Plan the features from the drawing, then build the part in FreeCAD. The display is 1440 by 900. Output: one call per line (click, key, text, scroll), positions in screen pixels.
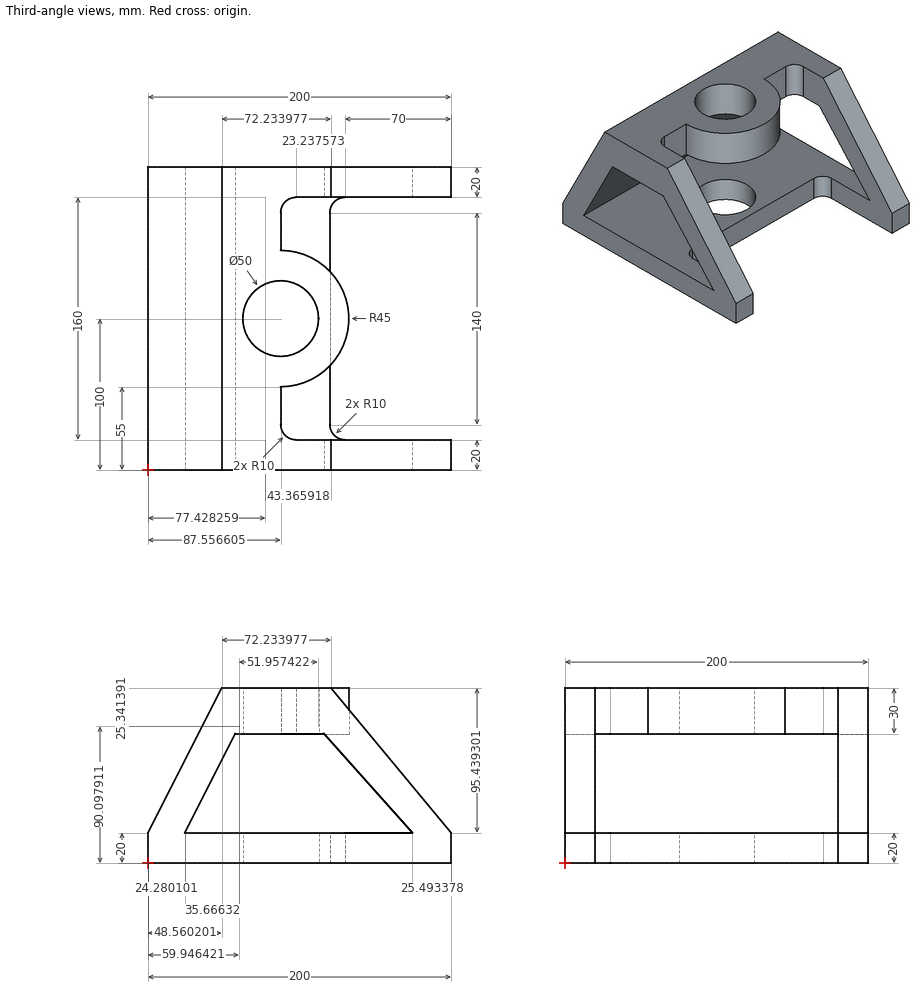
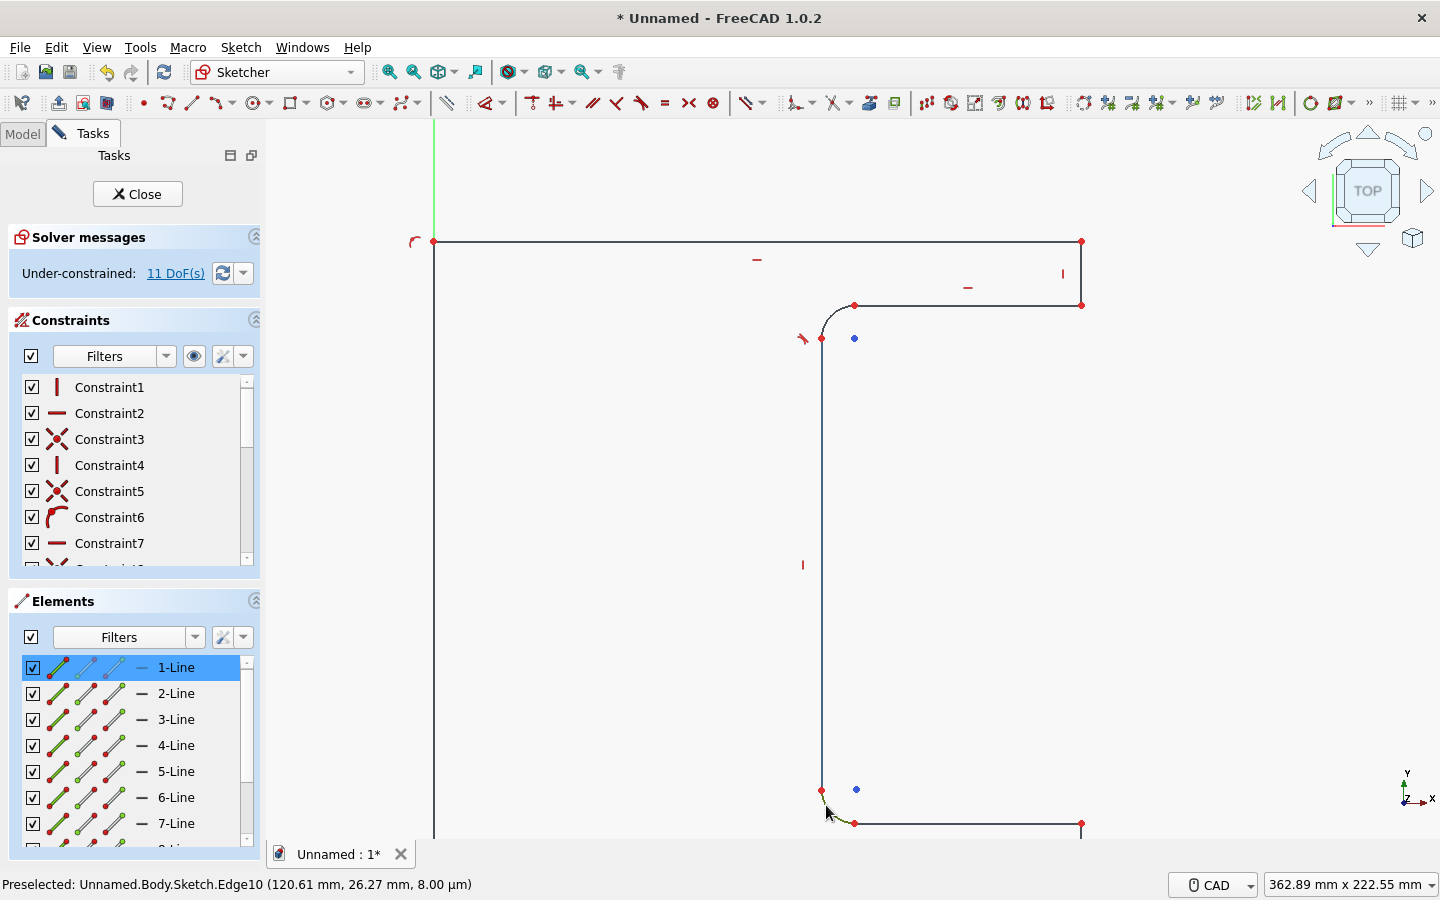
click(642, 104)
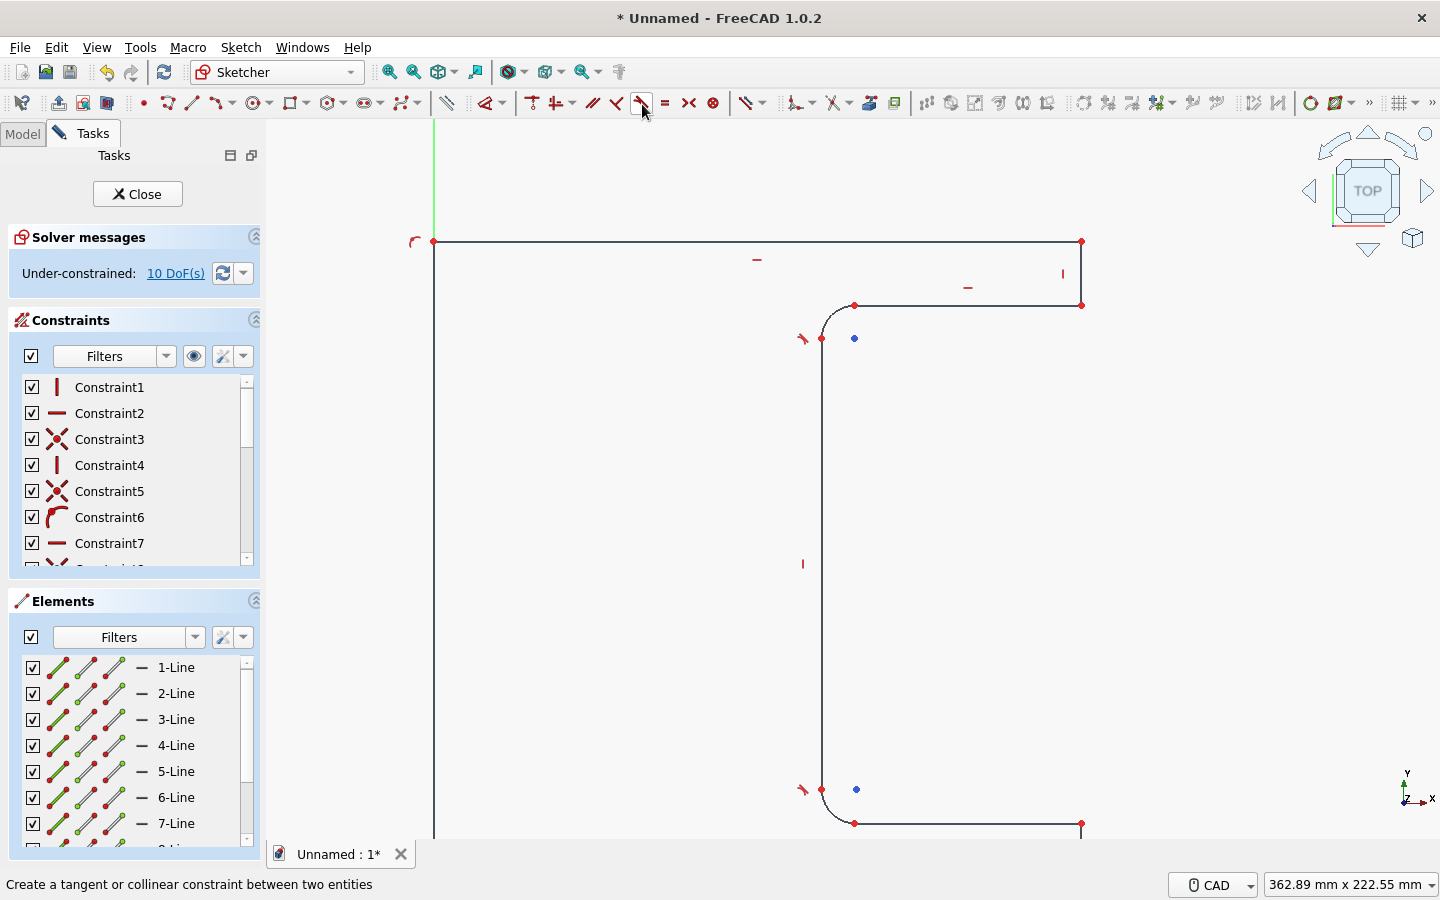
click(923, 306)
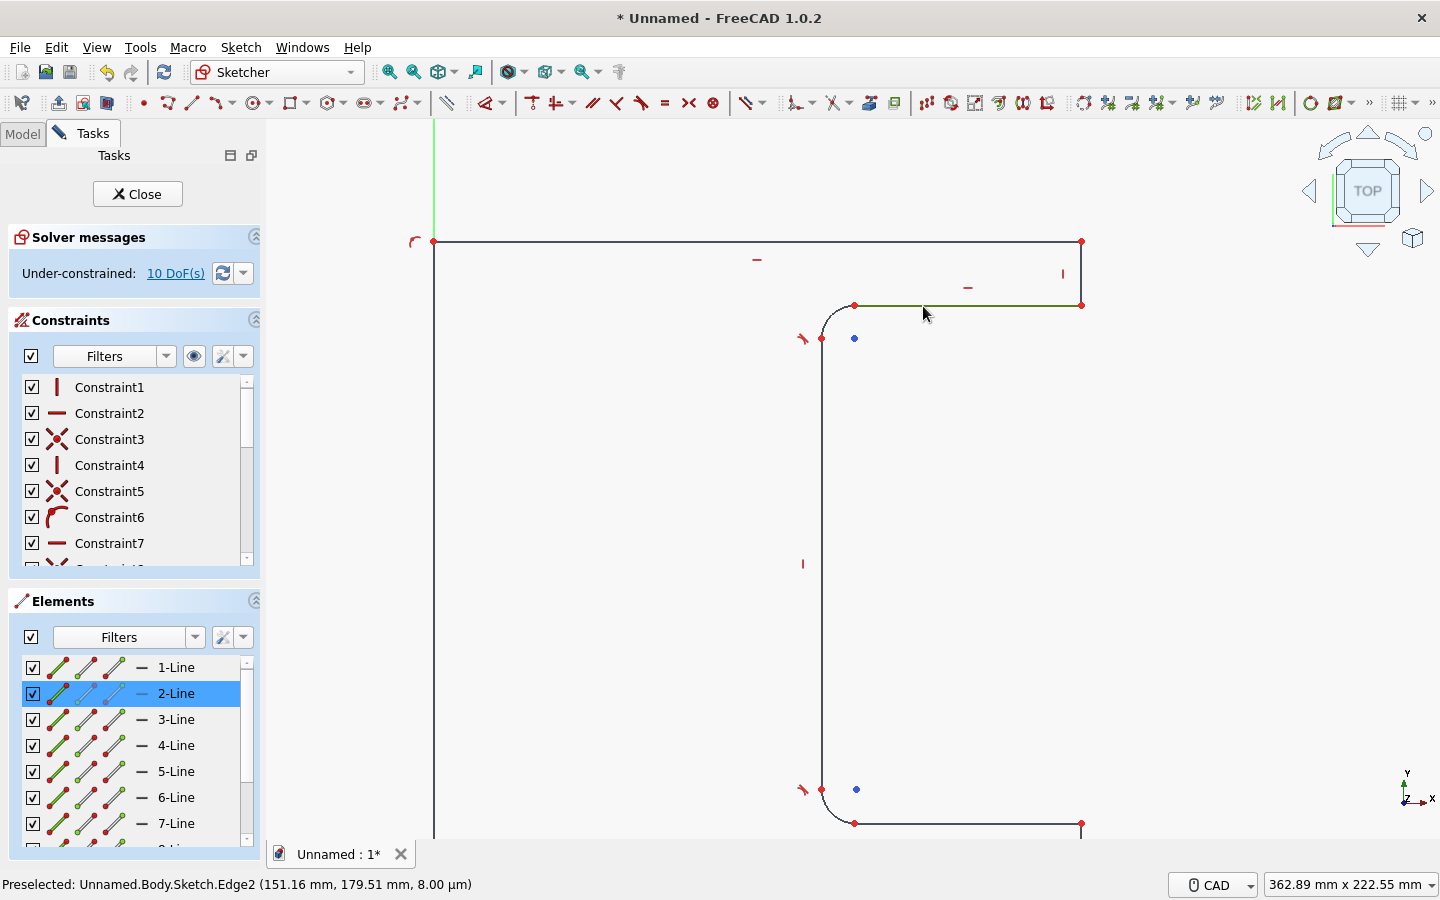
click(840, 309)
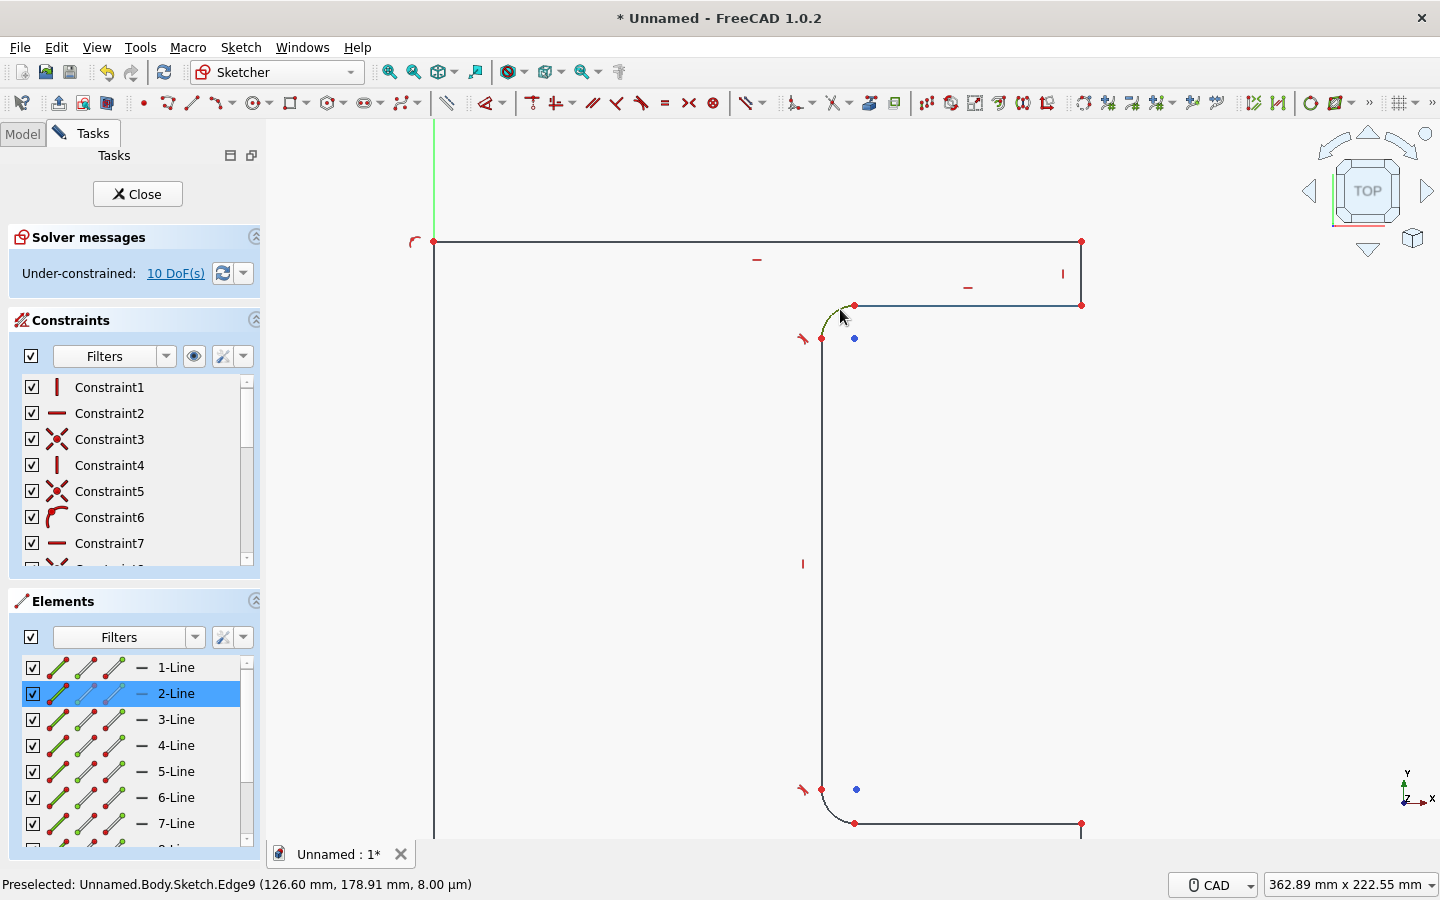
click(642, 104)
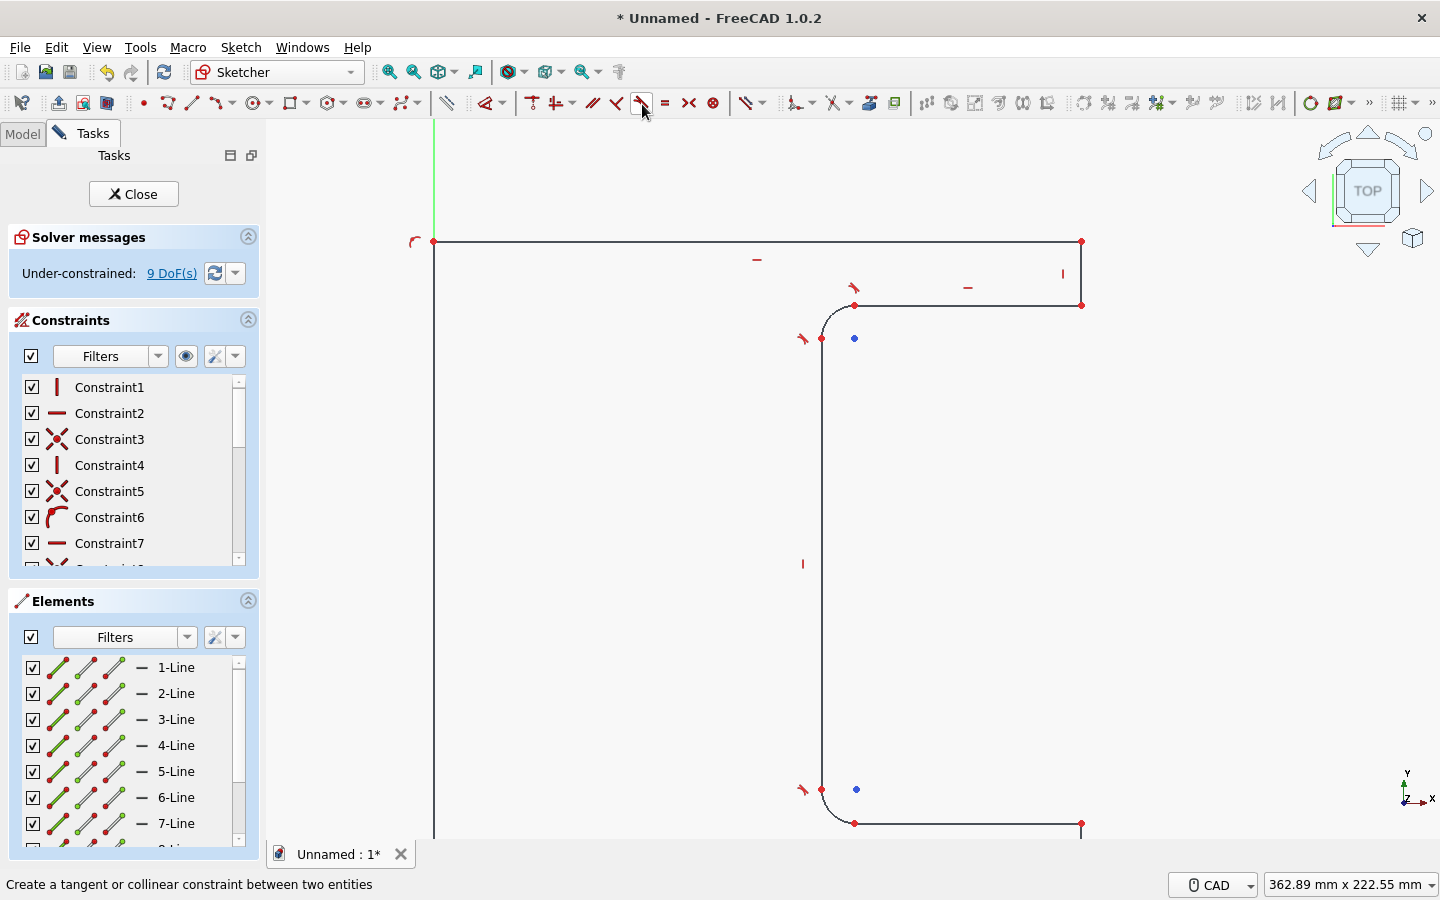
scroll(839, 308, down, 2)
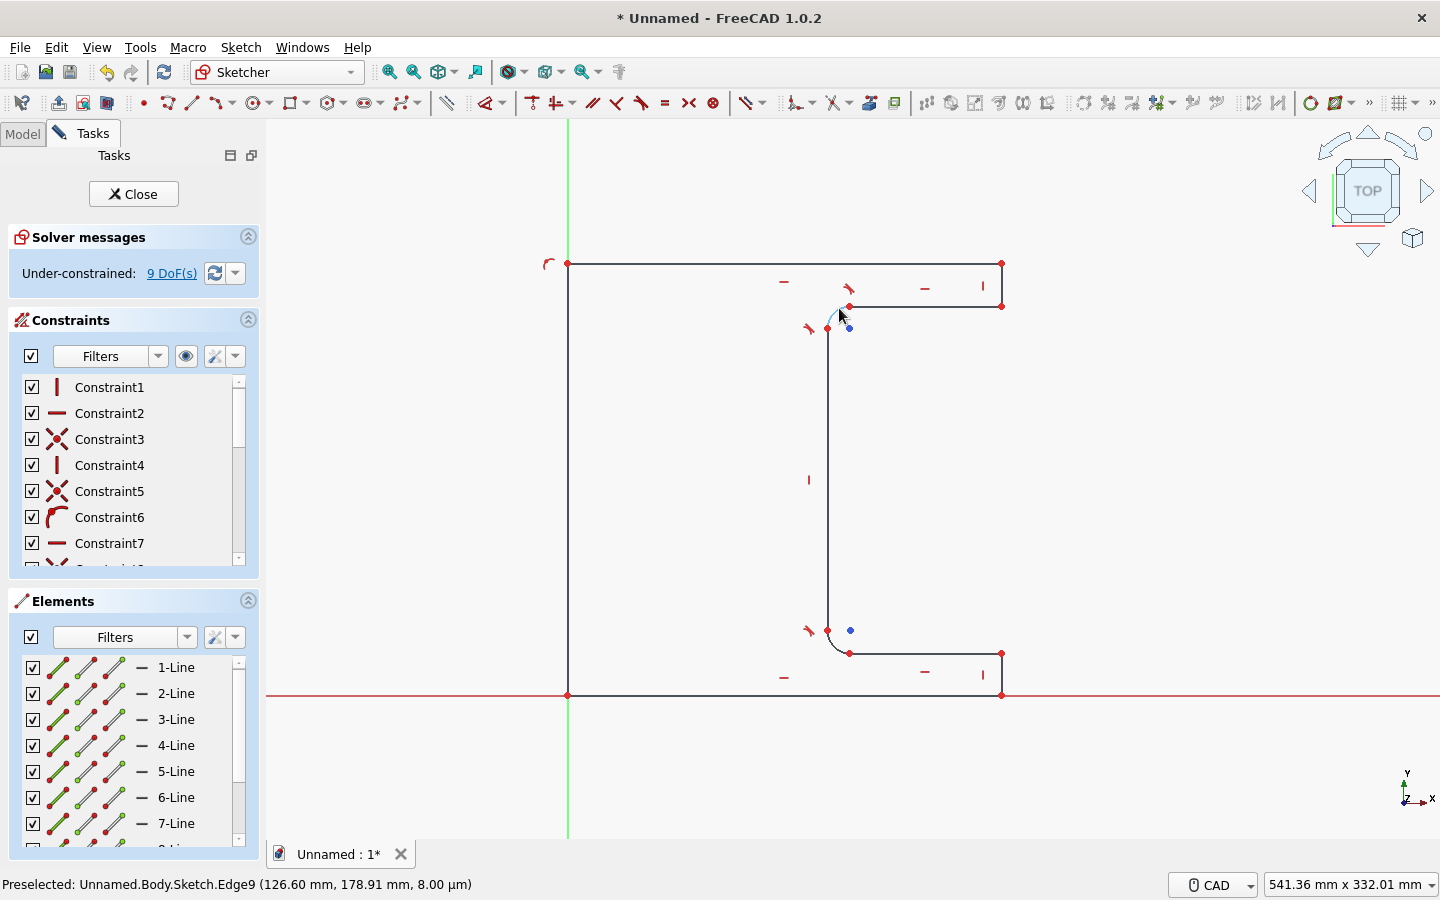
click(956, 654)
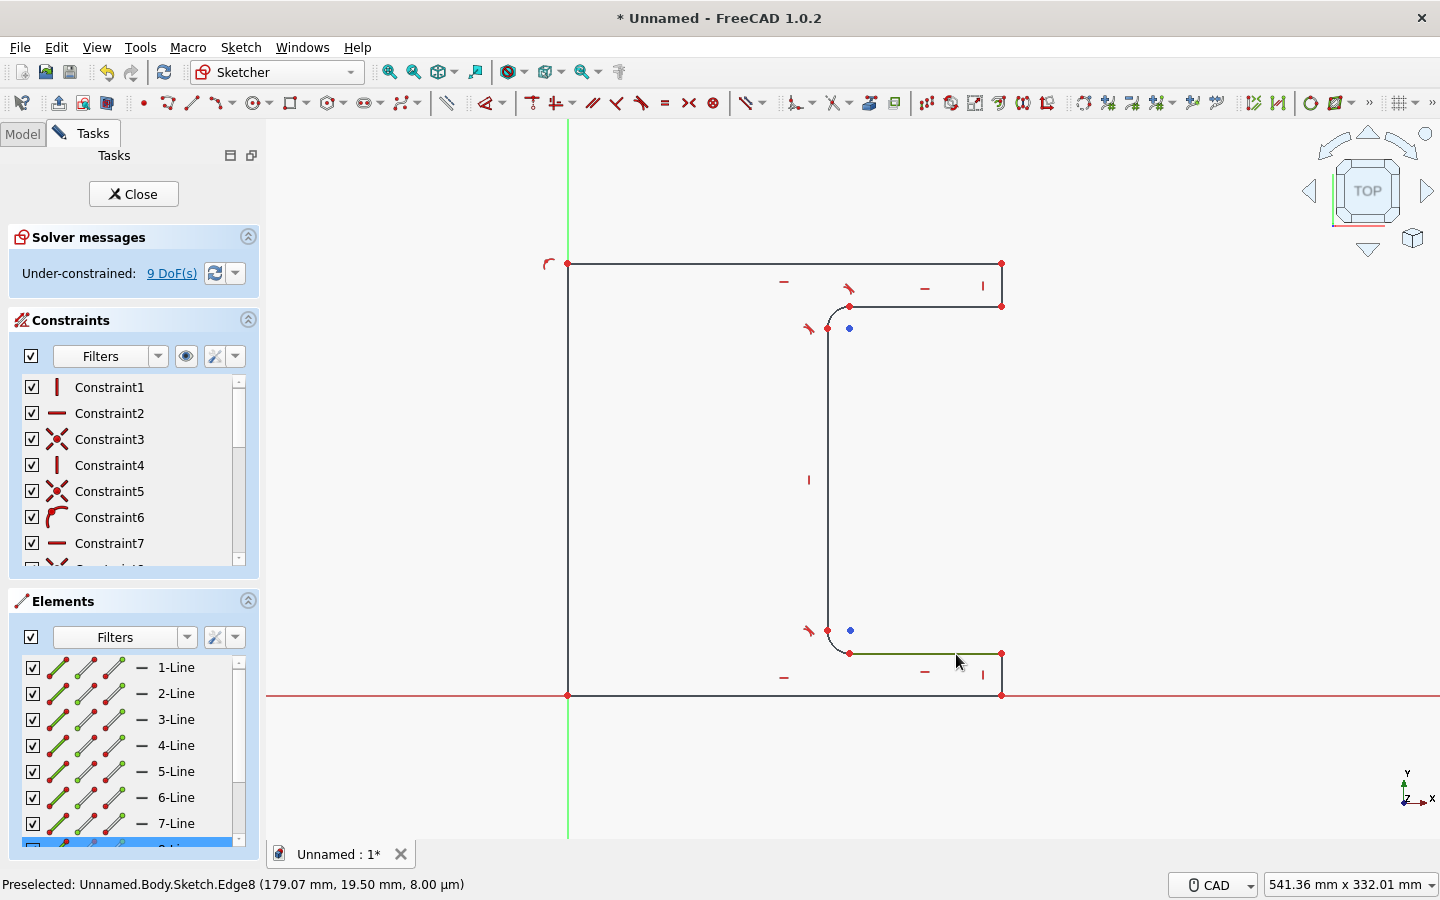
scroll(830, 641, up, 2)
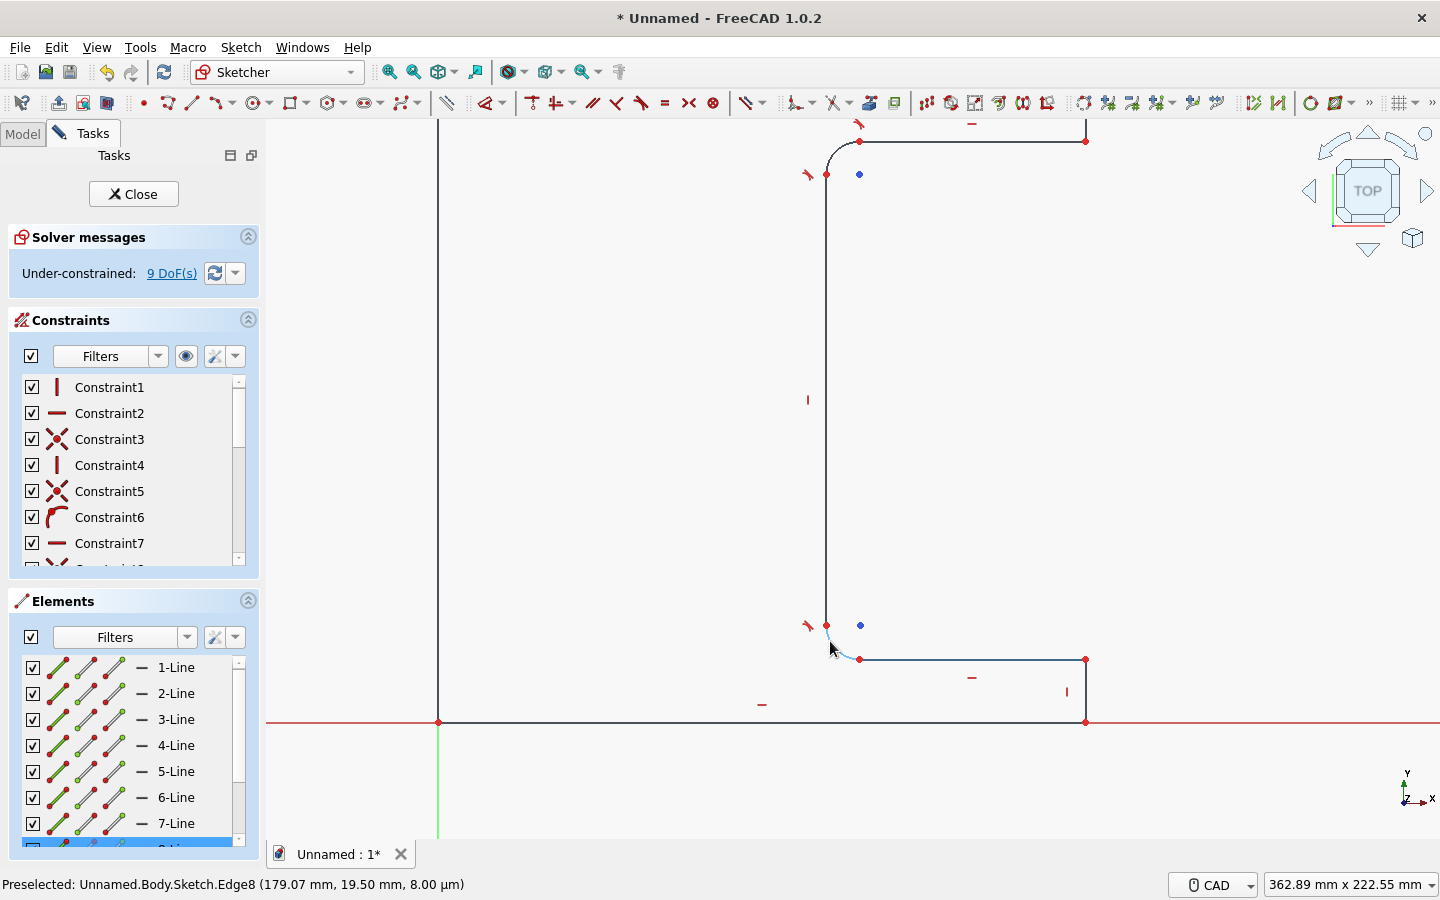
click(830, 640)